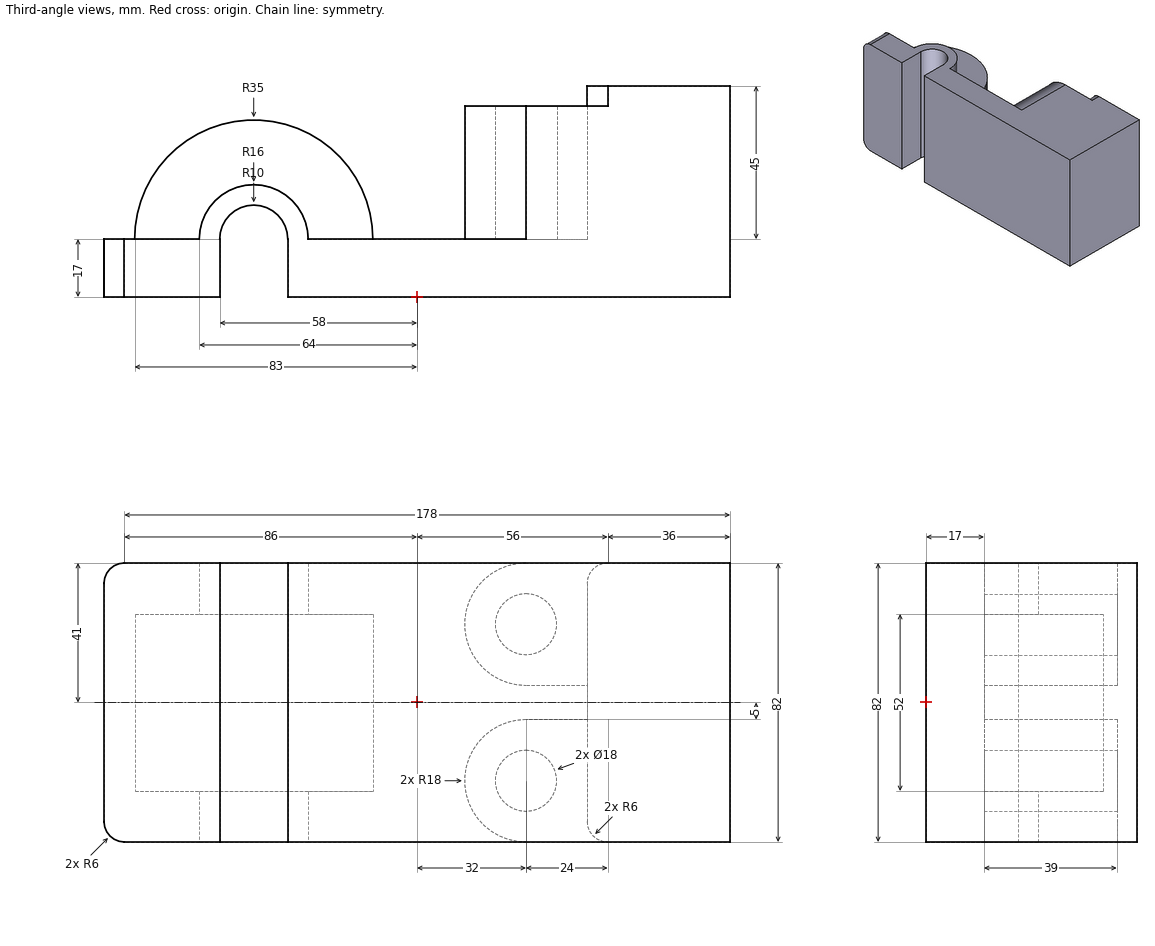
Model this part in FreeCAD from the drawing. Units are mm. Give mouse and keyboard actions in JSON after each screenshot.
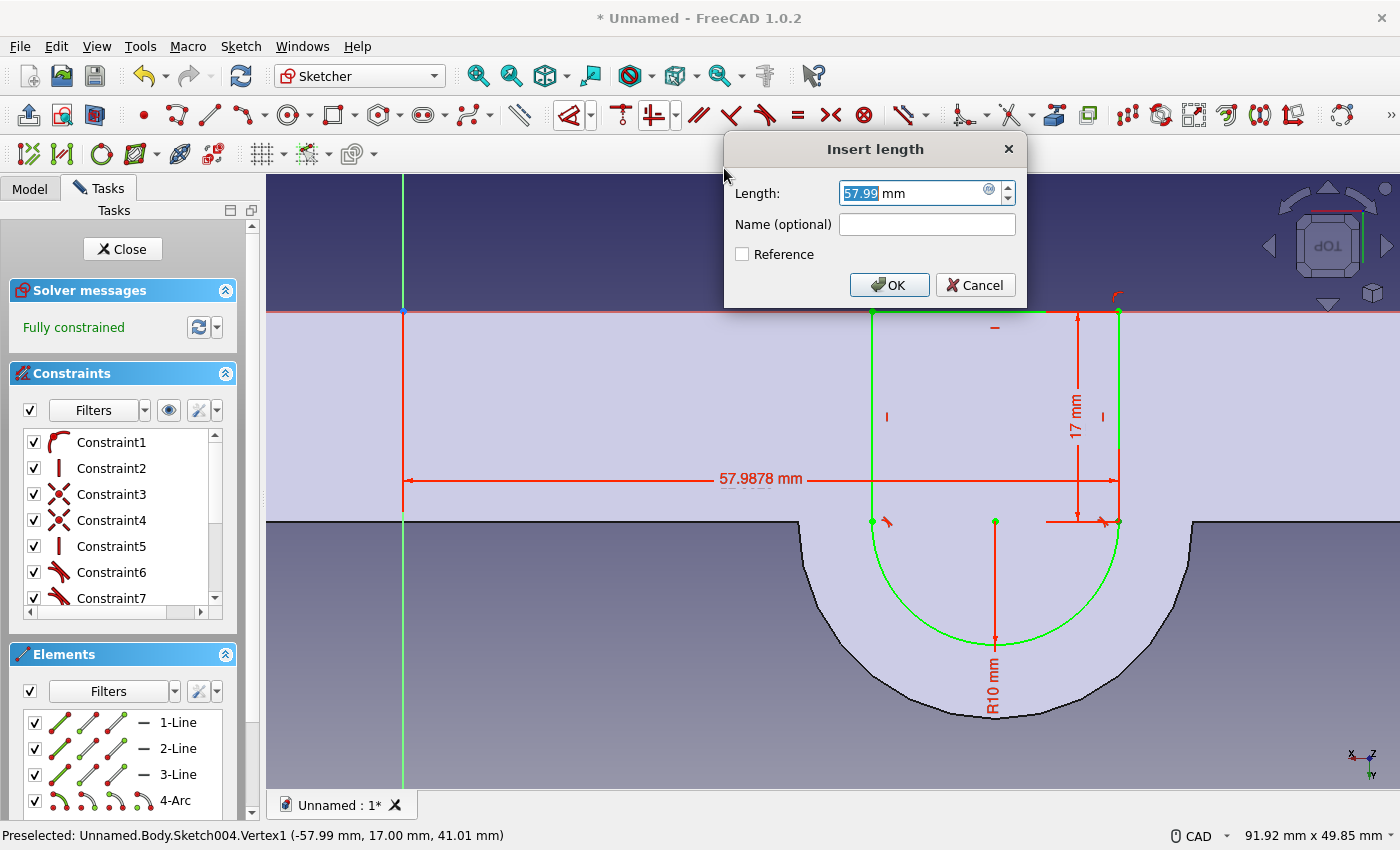
{"action": "type", "text": "58"}
{"action": "key", "text": "Return"}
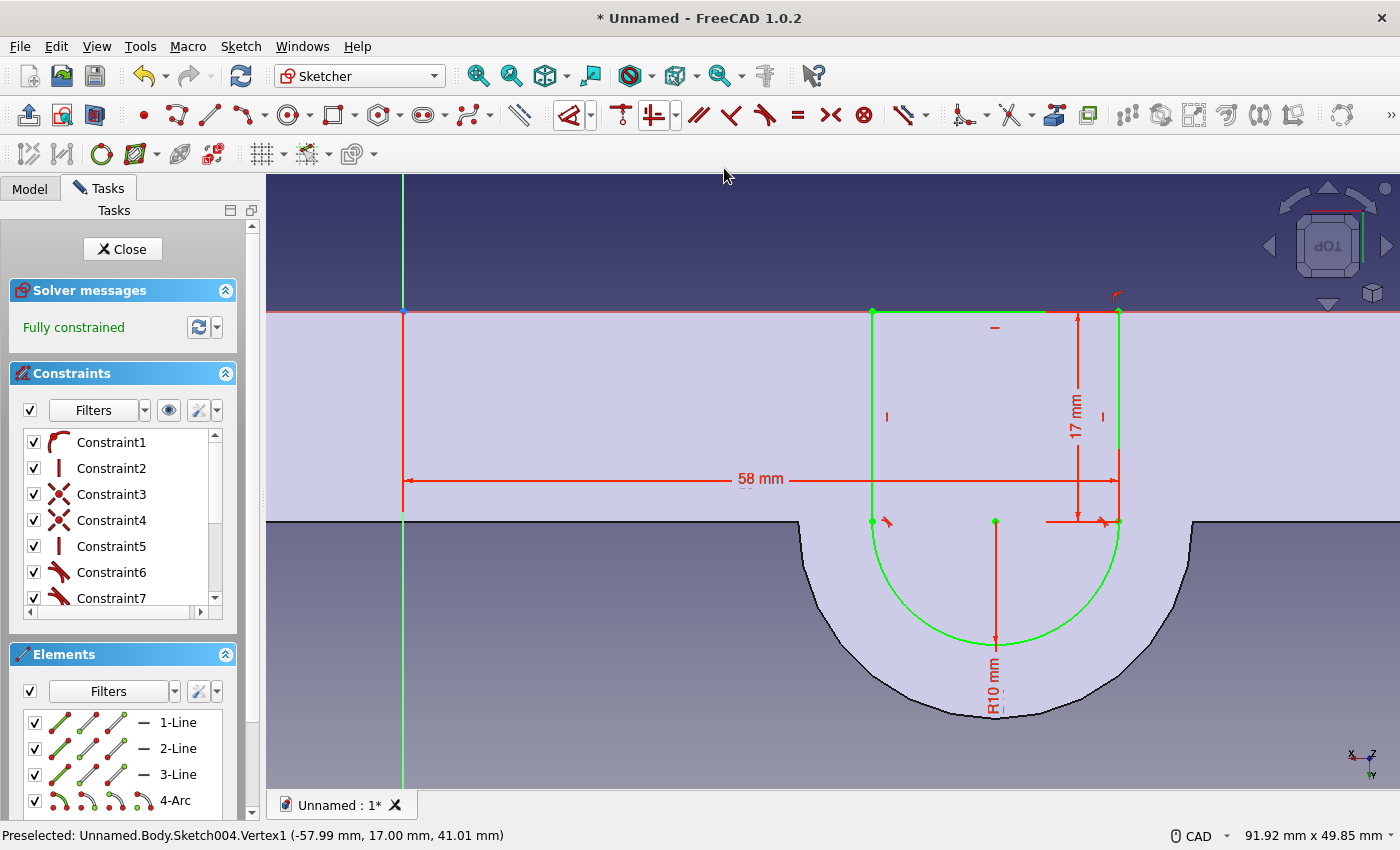
{"action": "left_click", "coordinate": [123, 249]}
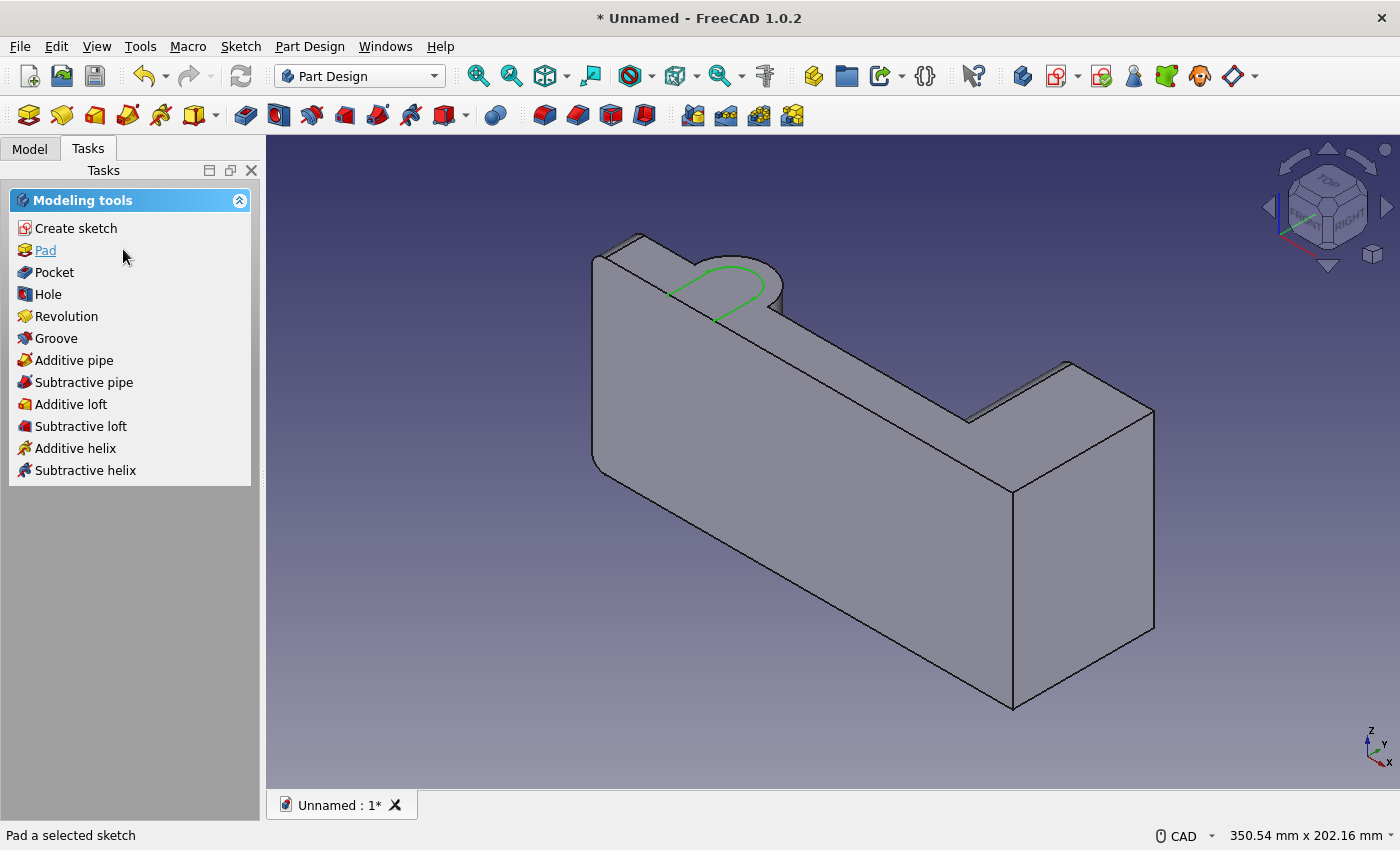
{"action": "left_click", "coordinate": [246, 116]}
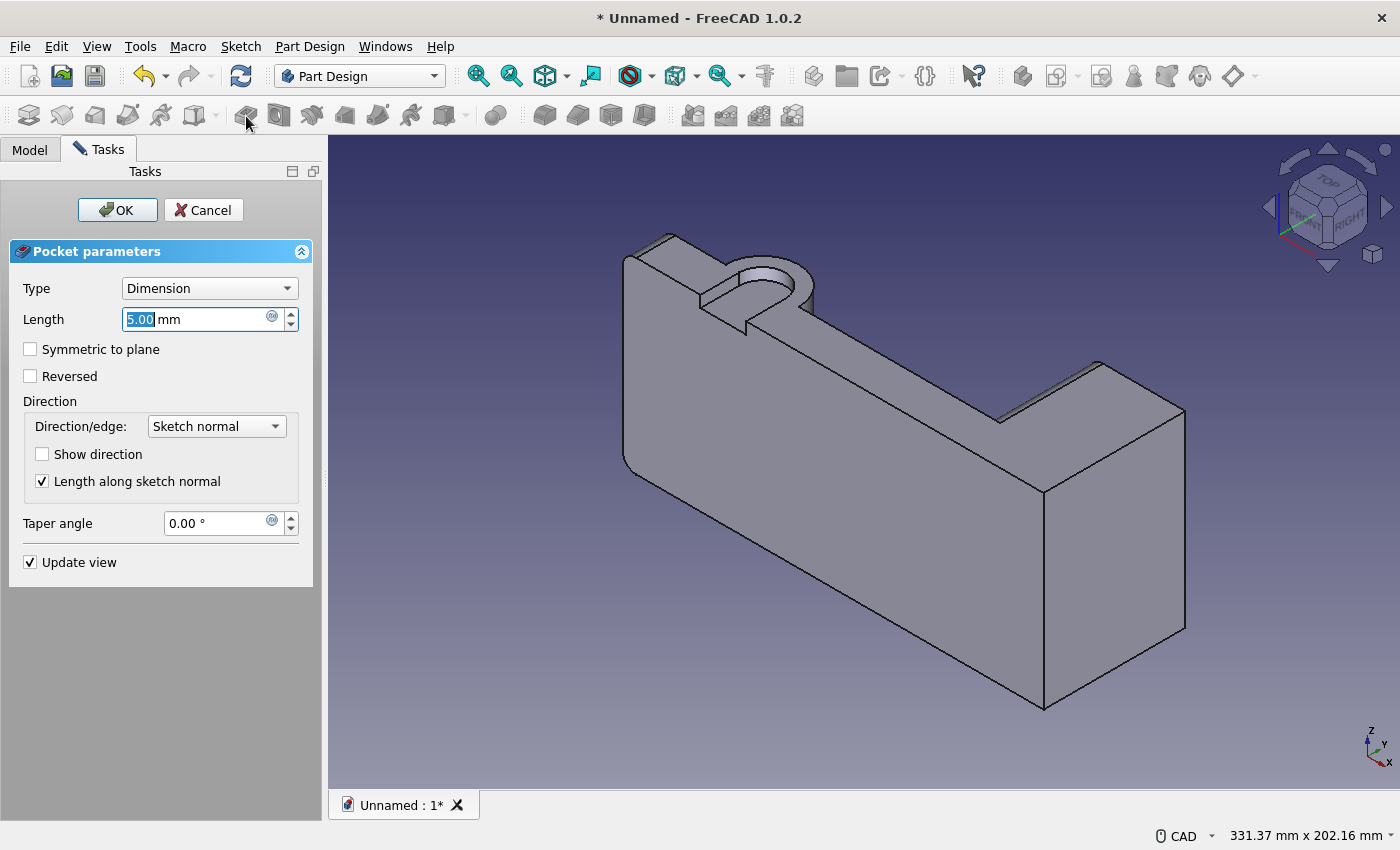
{"action": "type", "text": "82"}
{"action": "key", "text": "Tab"}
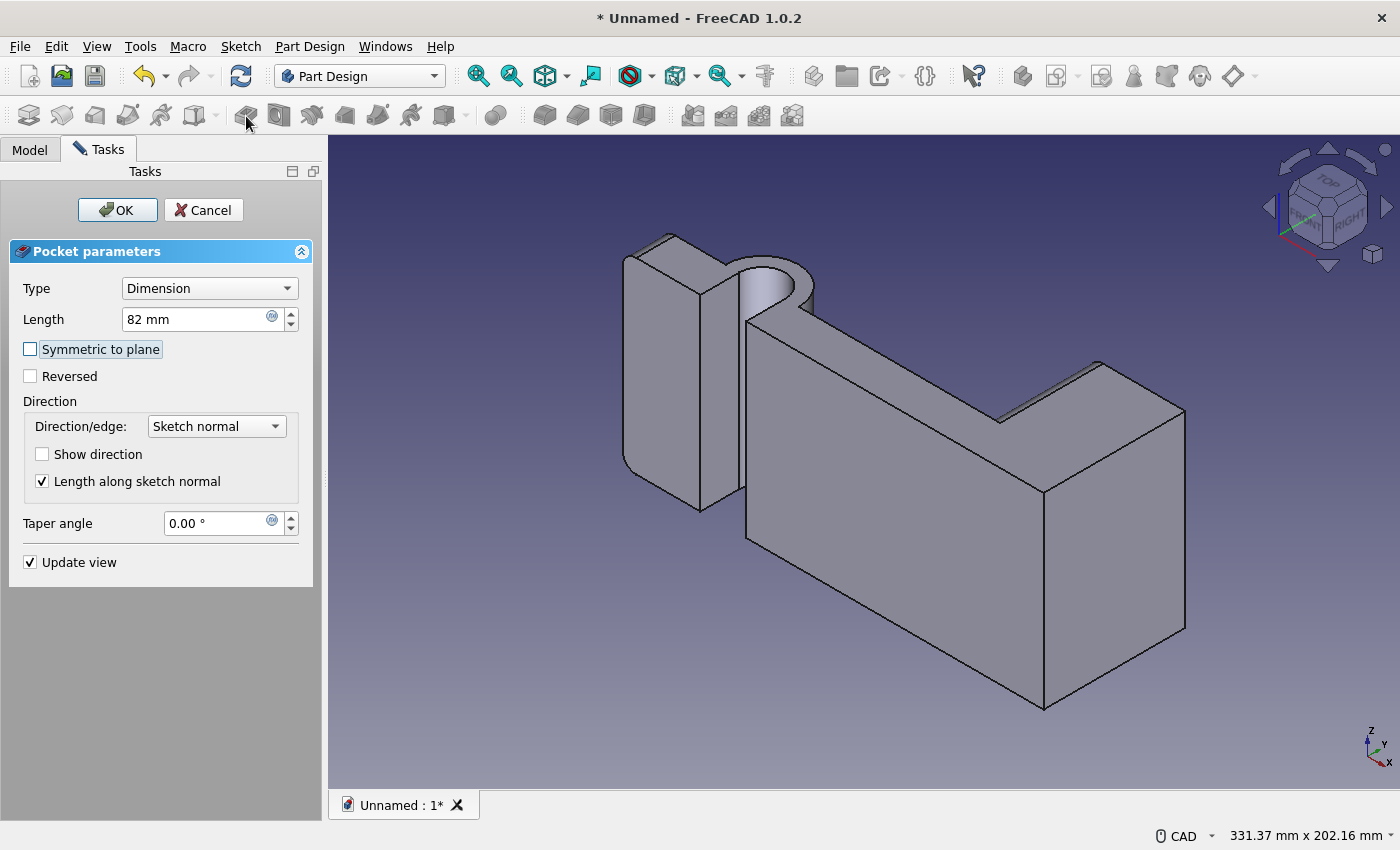
{"action": "left_click", "coordinate": [118, 210]}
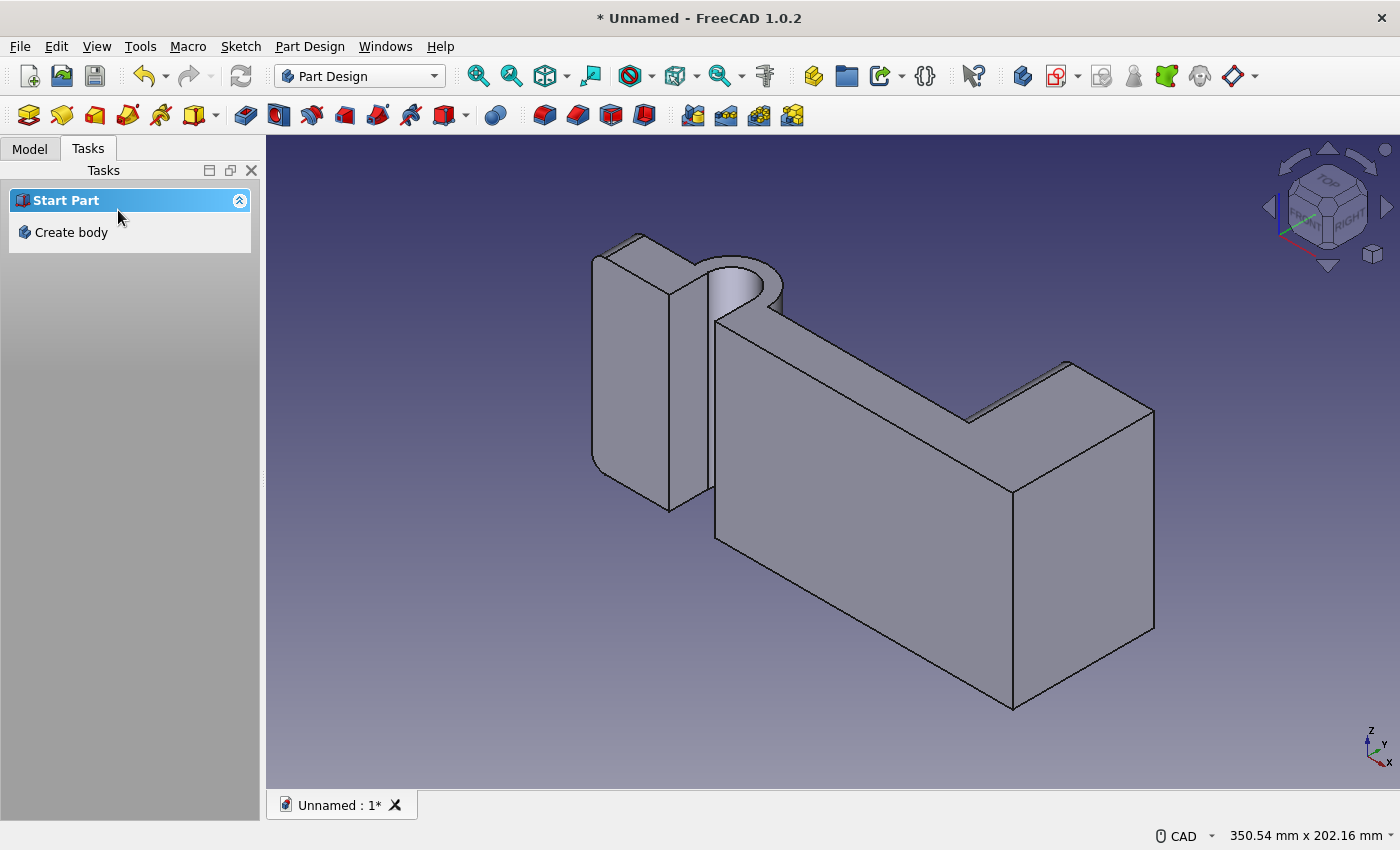
{"action": "key", "text": "4"}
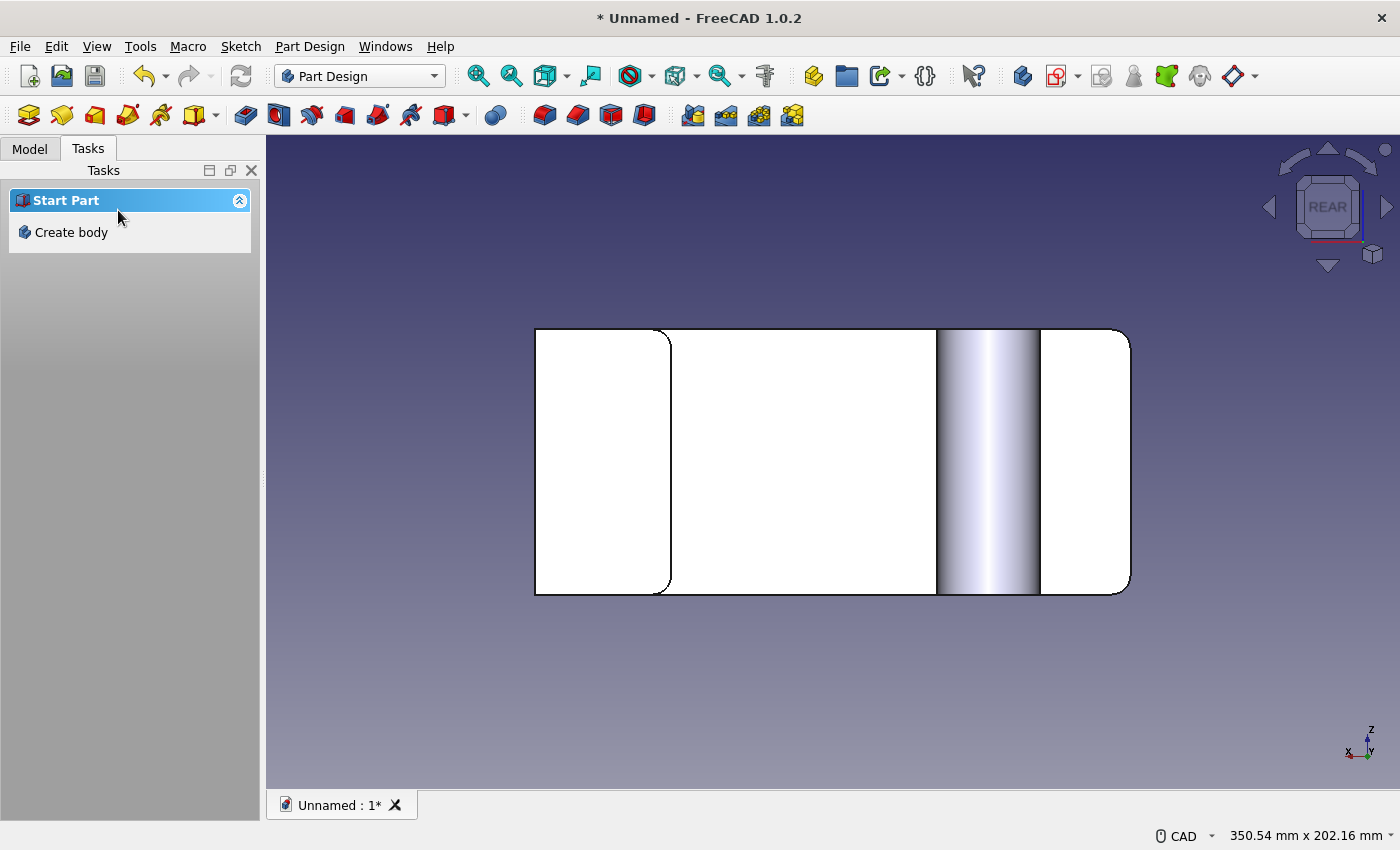
{"action": "left_click", "coordinate": [794, 461]}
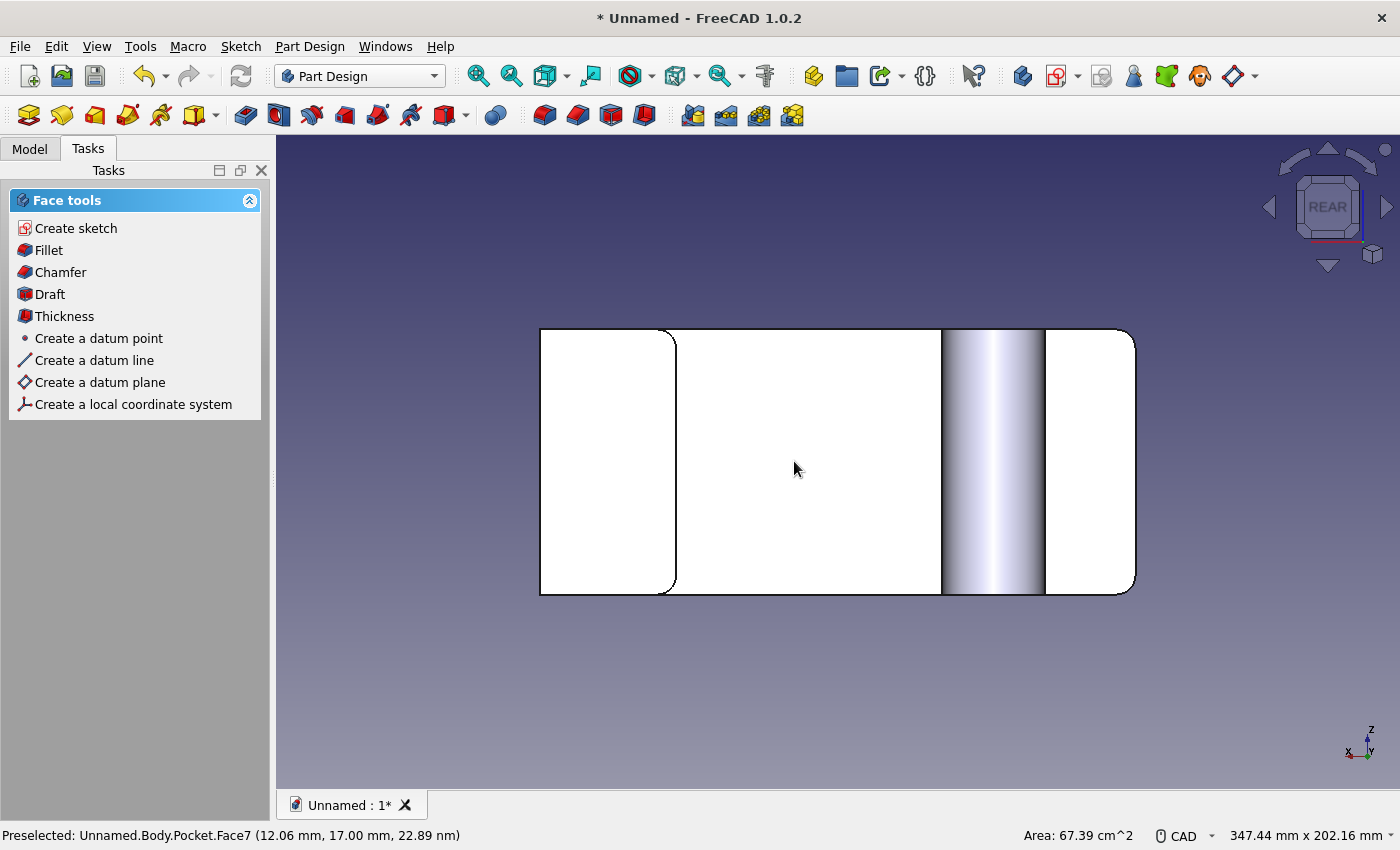
{"action": "left_click", "coordinate": [1056, 76]}